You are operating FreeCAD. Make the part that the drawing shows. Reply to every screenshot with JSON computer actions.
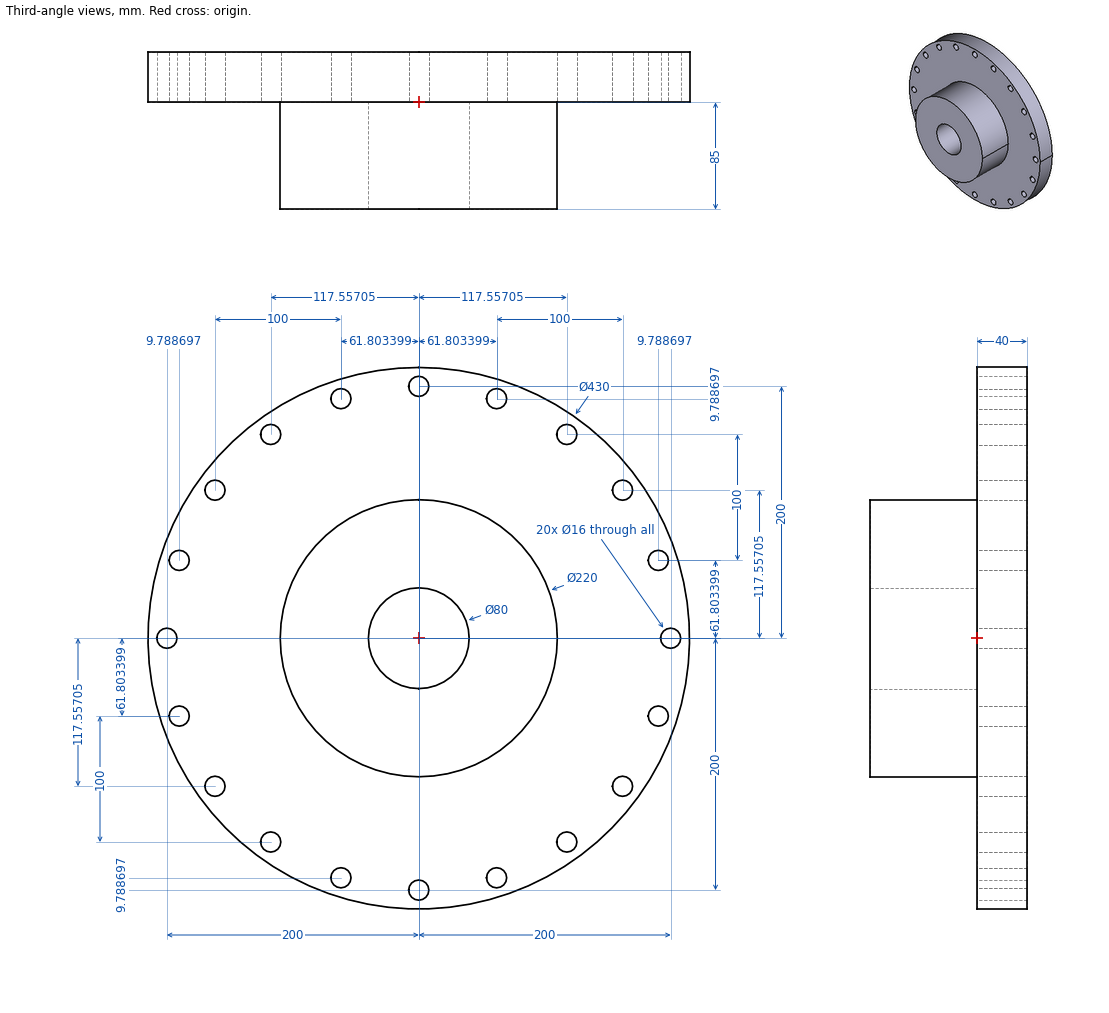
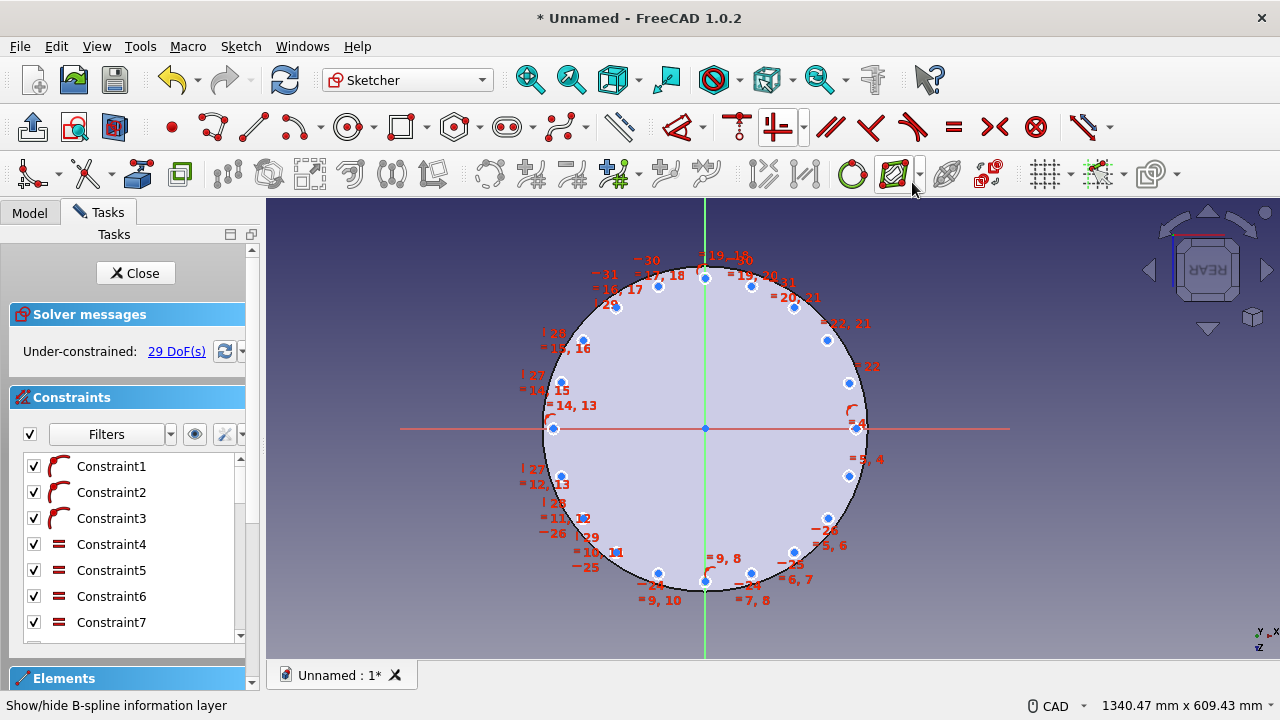
{"action": "left_click", "coordinate": [828, 519]}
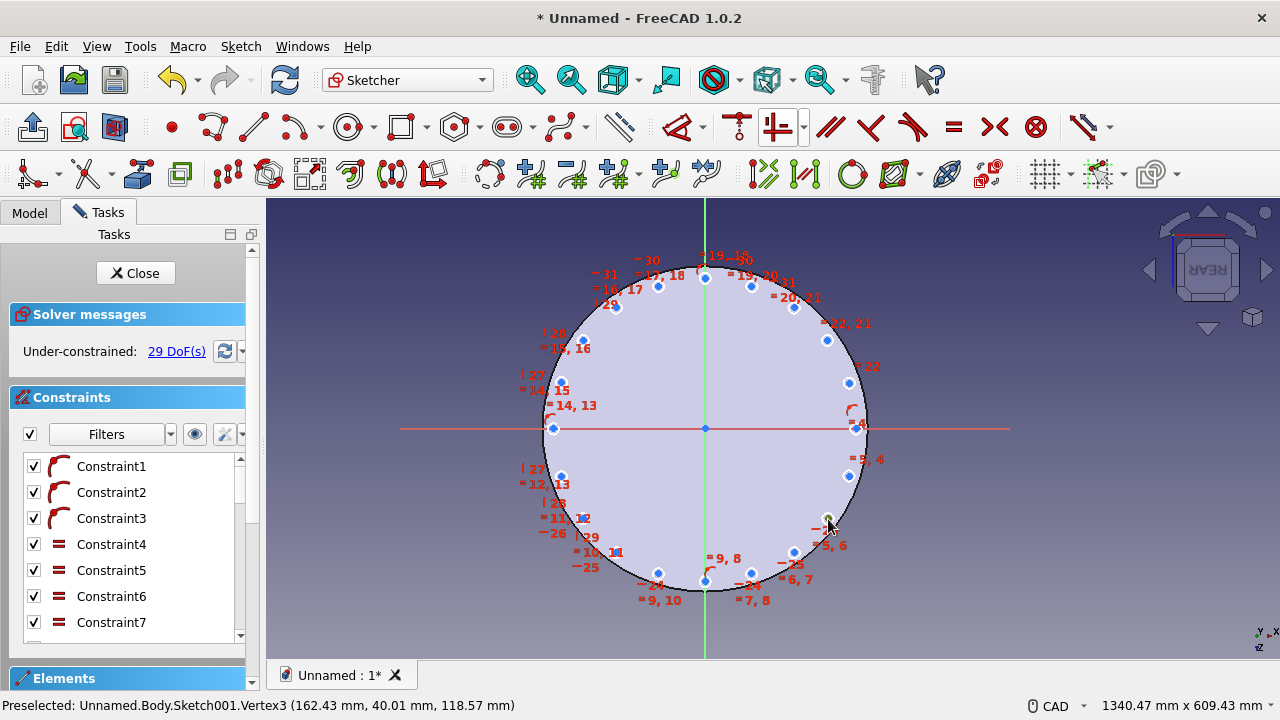
{"action": "left_click", "coordinate": [828, 340]}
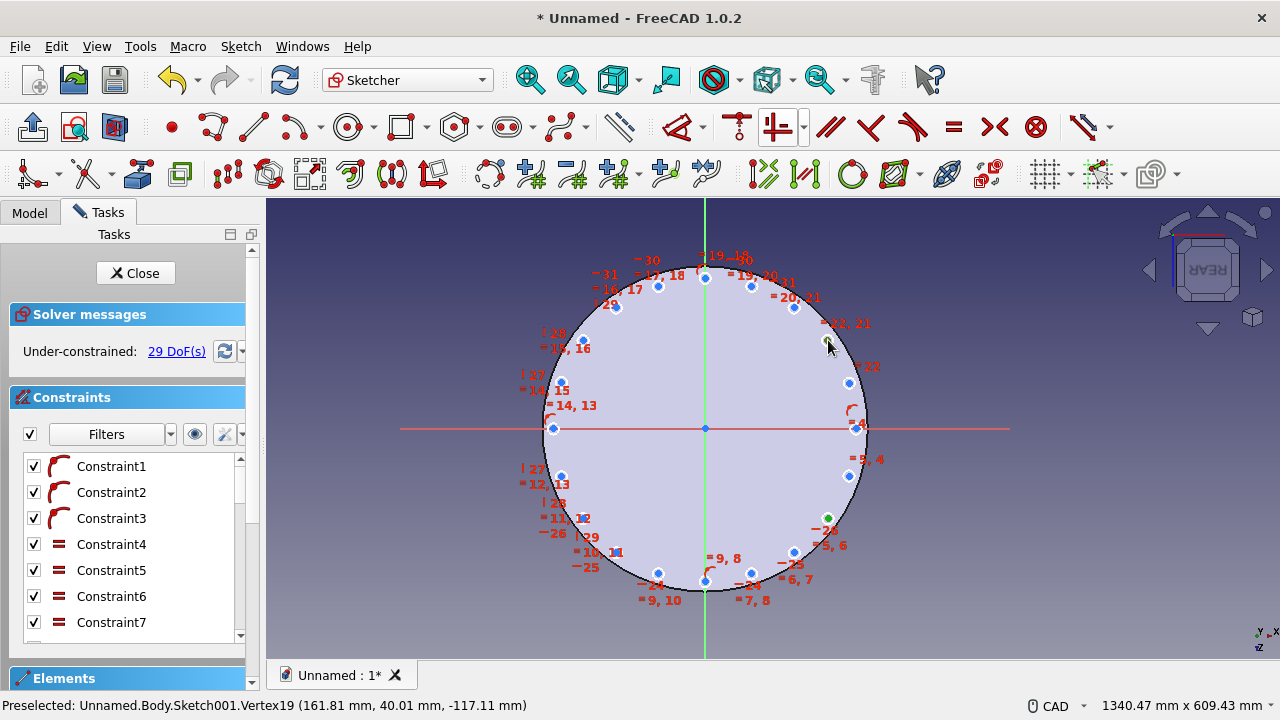
{"action": "key", "text": "v"}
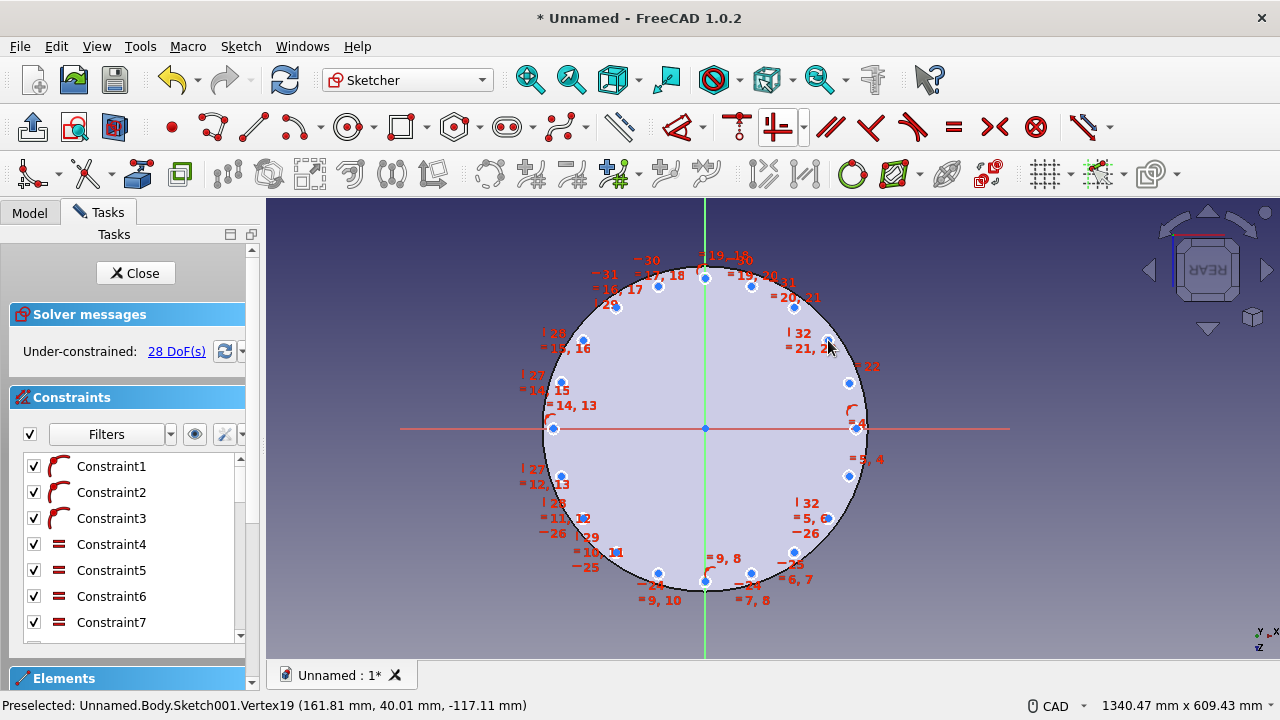
{"action": "left_click", "coordinate": [849, 476]}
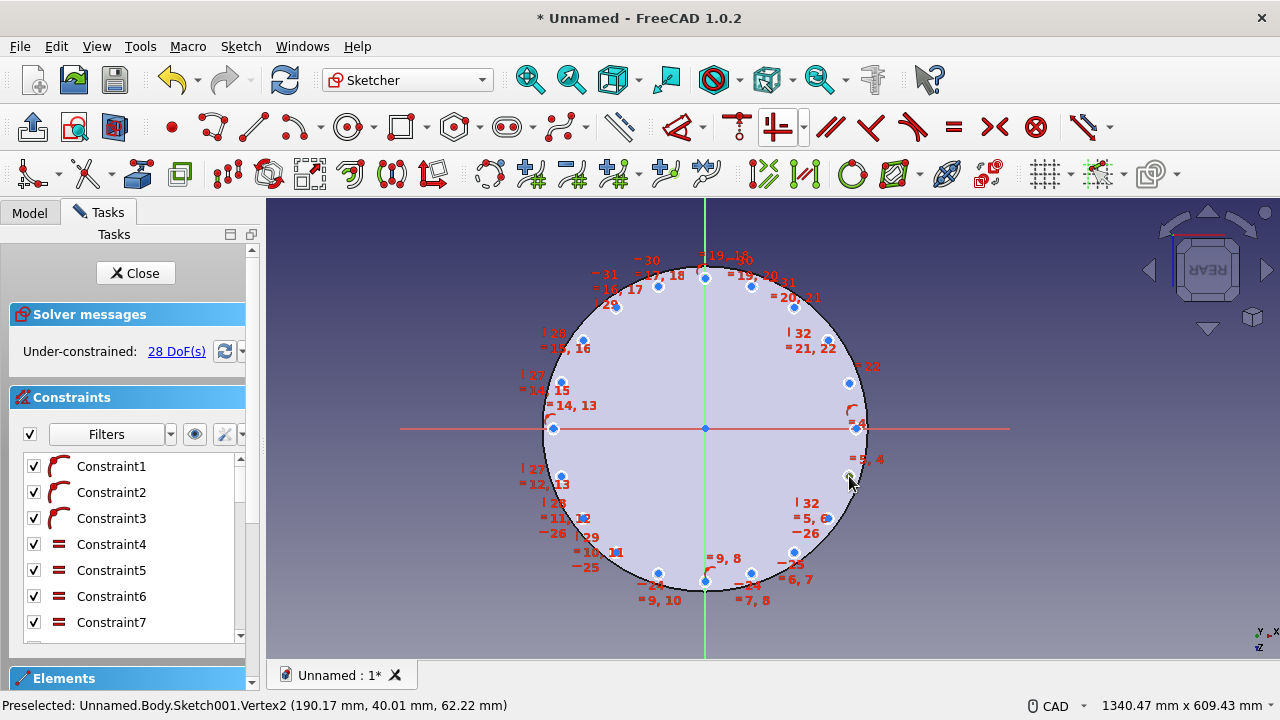
{"action": "left_click", "coordinate": [849, 383]}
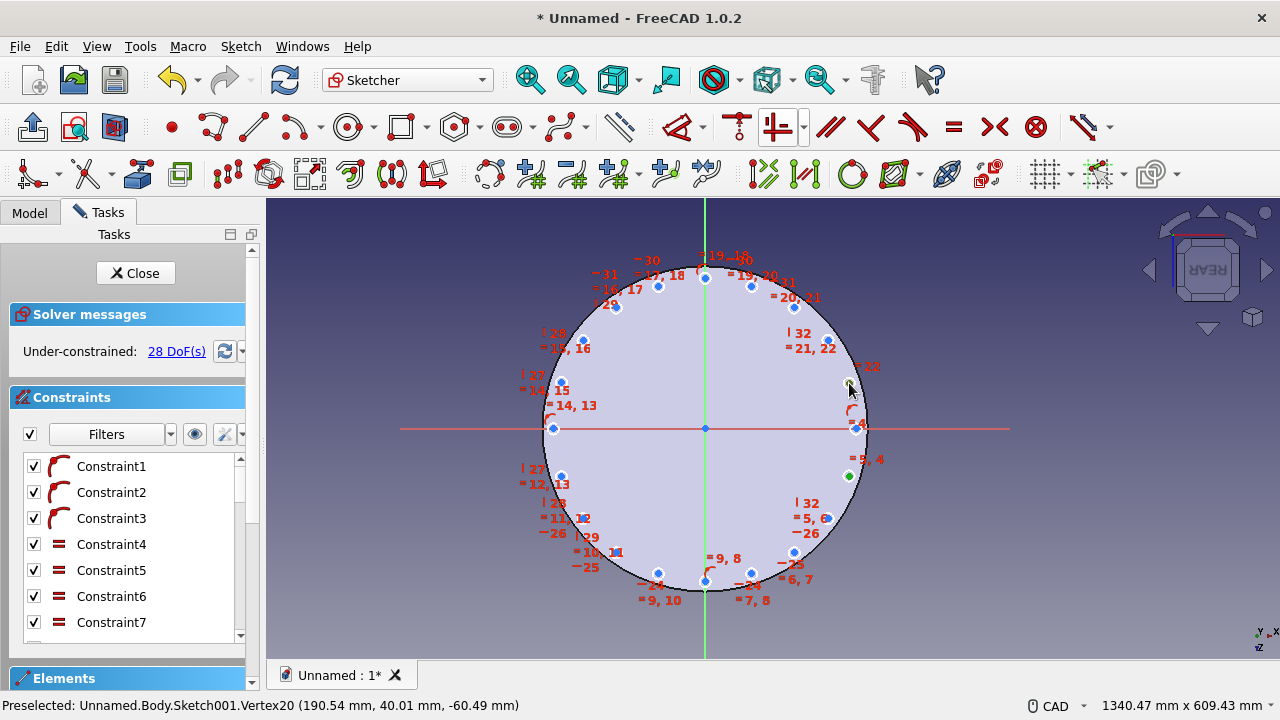
{"action": "left_click", "coordinate": [804, 128]}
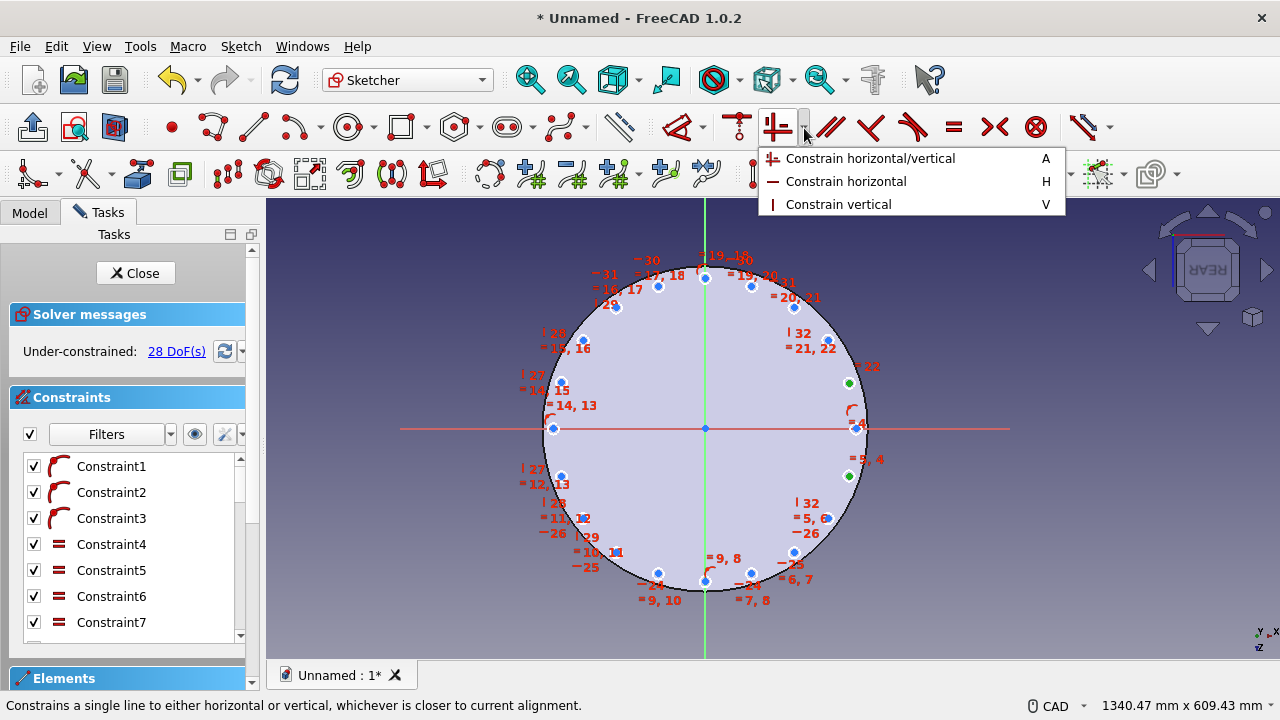
{"action": "left_click", "coordinate": [912, 204]}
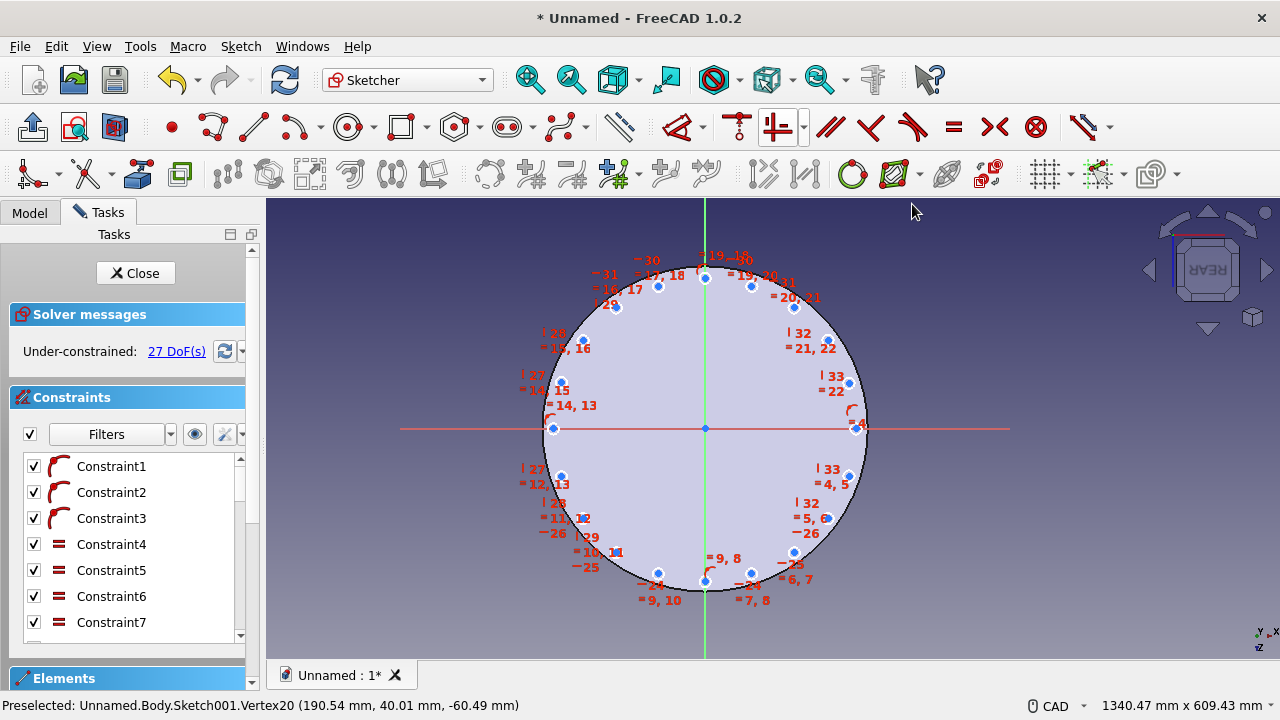
{"action": "key", "text": "d"}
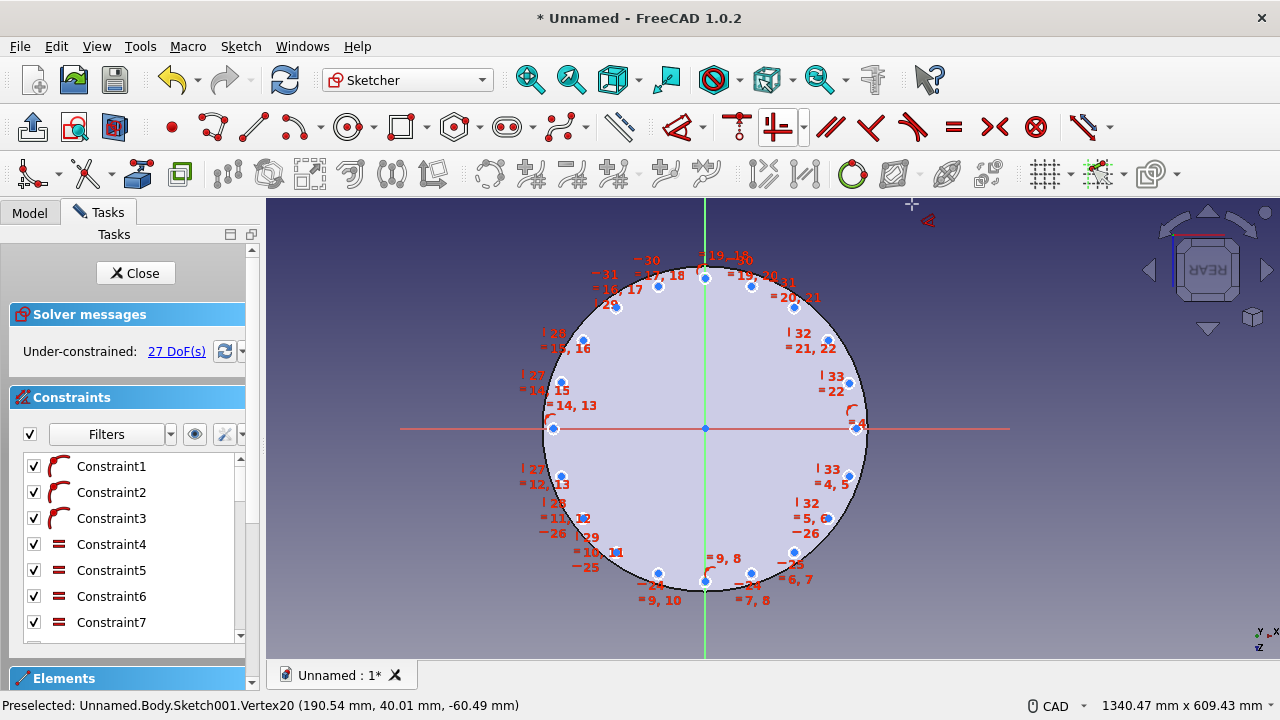
{"action": "scroll", "coordinate": [852, 433], "scroll_direction": "up", "scroll_amount": 6}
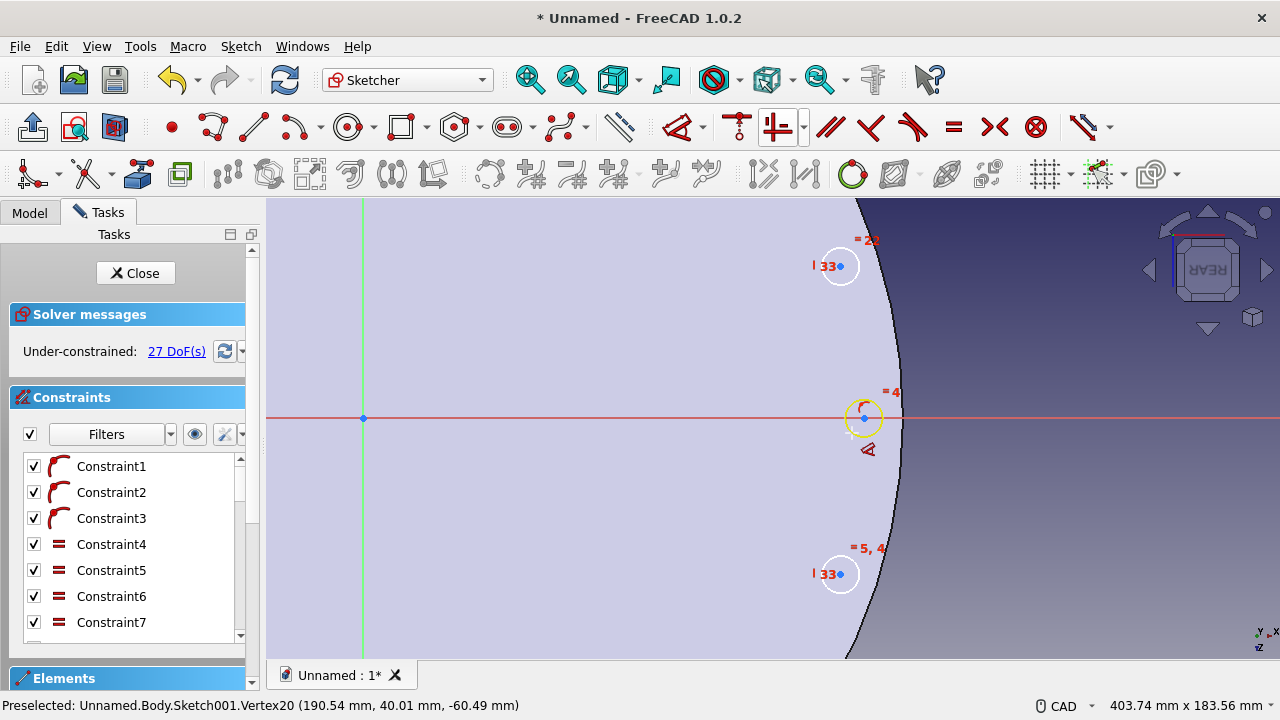
{"action": "left_click", "coordinate": [851, 432]}
{"action": "left_click", "coordinate": [829, 455]}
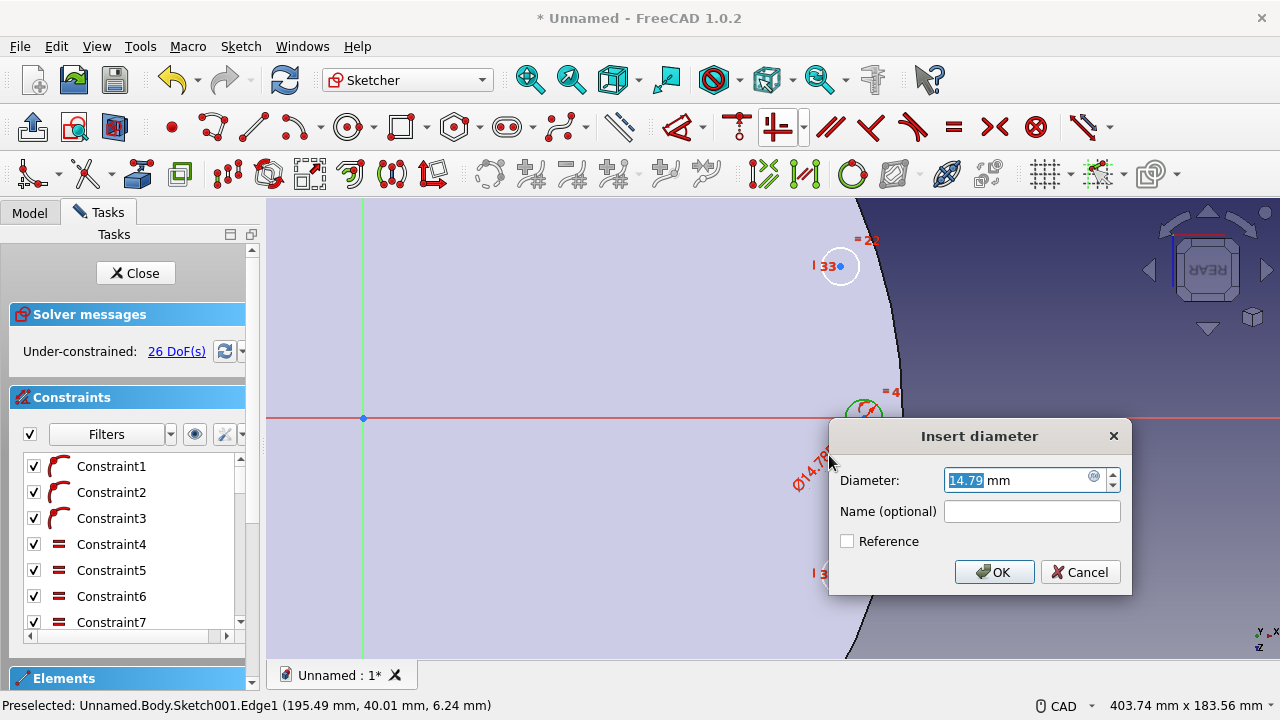
{"action": "type", "text": "16"}
{"action": "key", "text": "Return"}